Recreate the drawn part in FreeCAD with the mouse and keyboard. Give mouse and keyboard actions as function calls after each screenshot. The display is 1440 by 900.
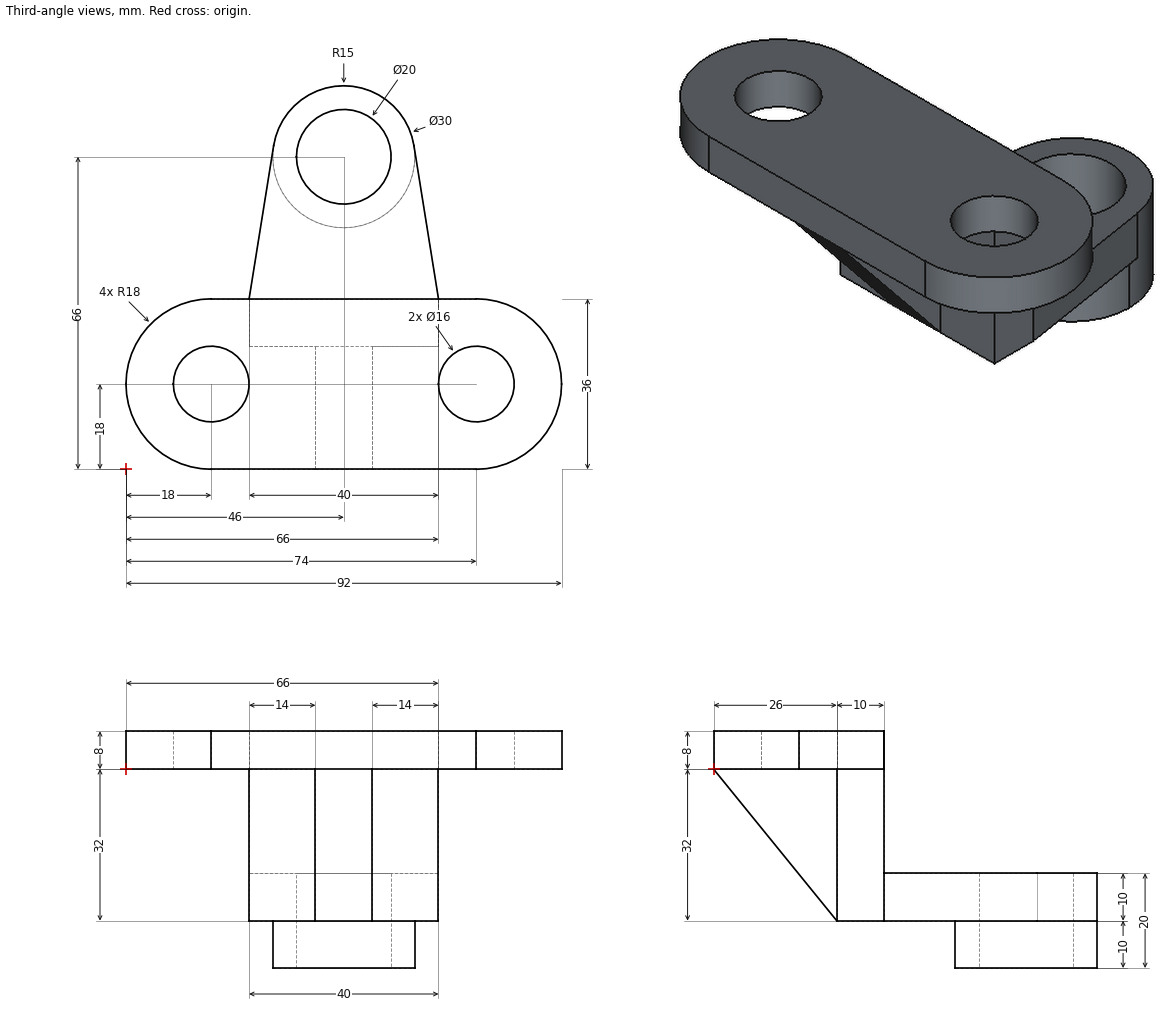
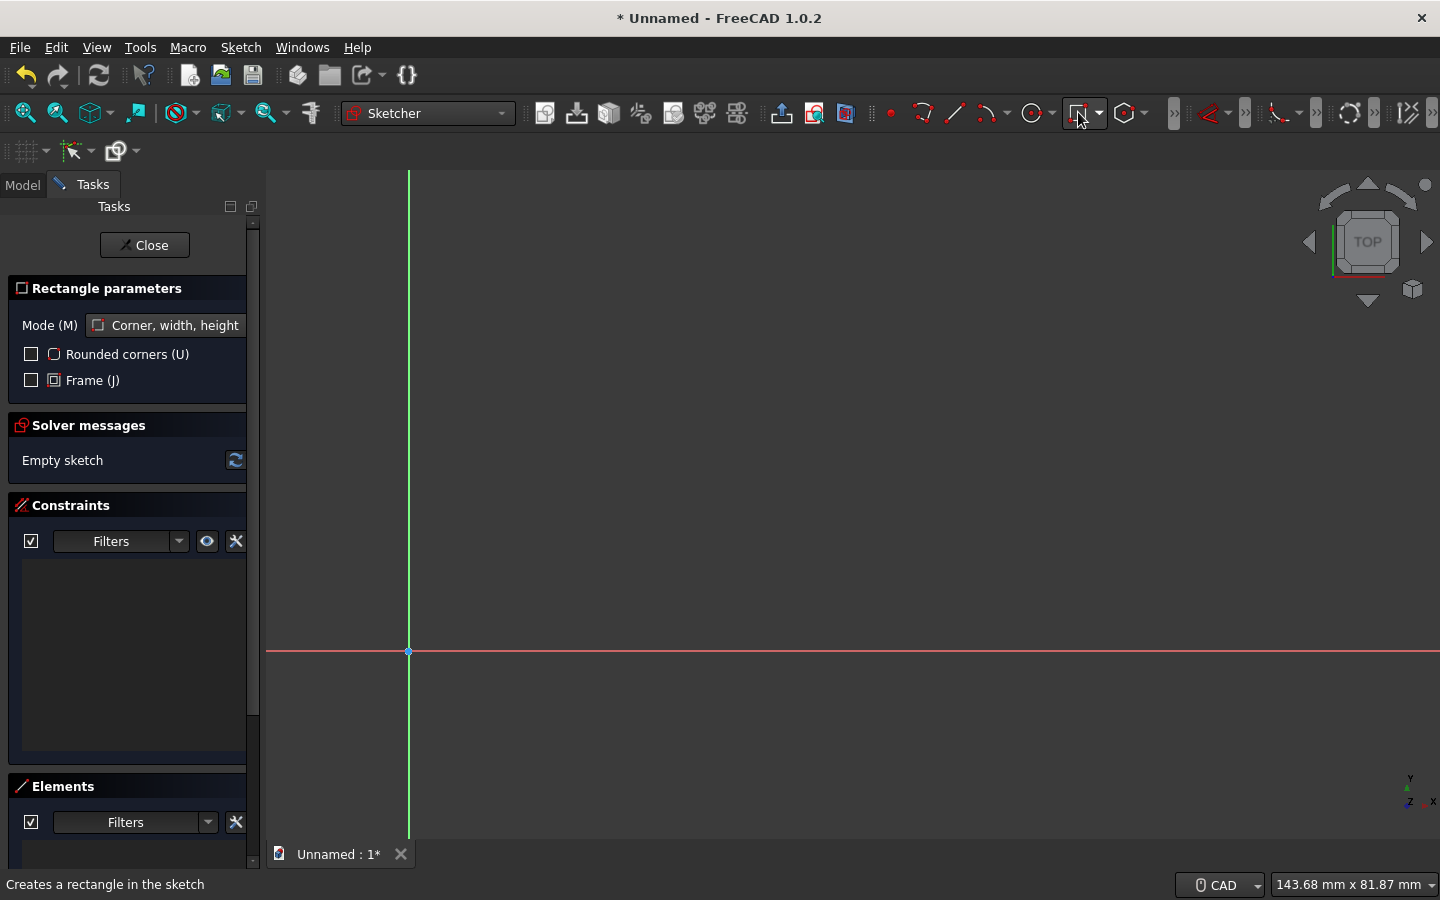
click(409, 651)
move(1160, 357)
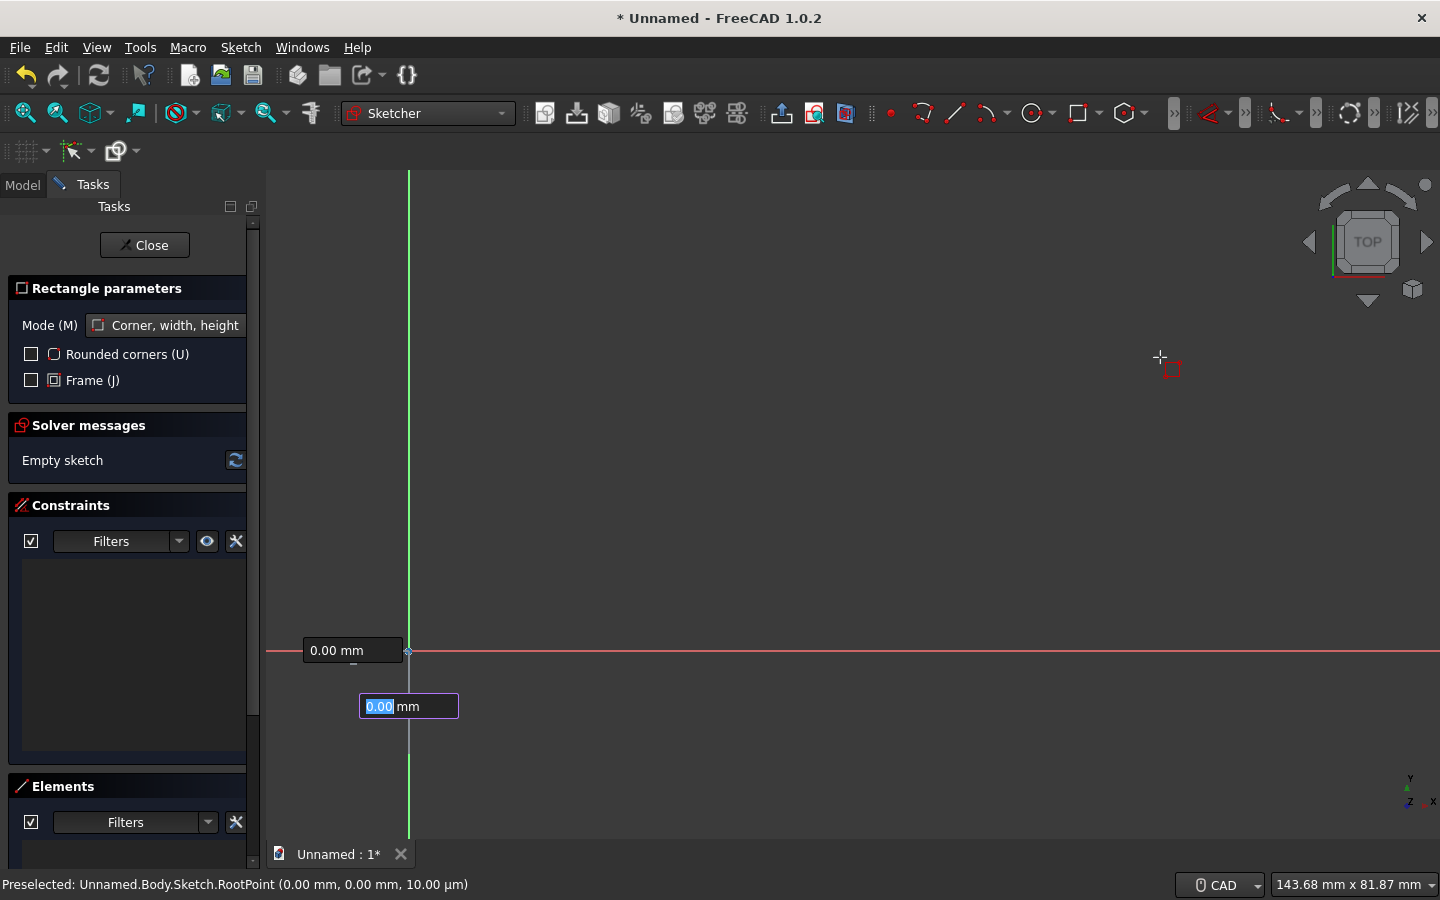
text(92)
key(Tab)
text(36)
key(Return)
key(Escape)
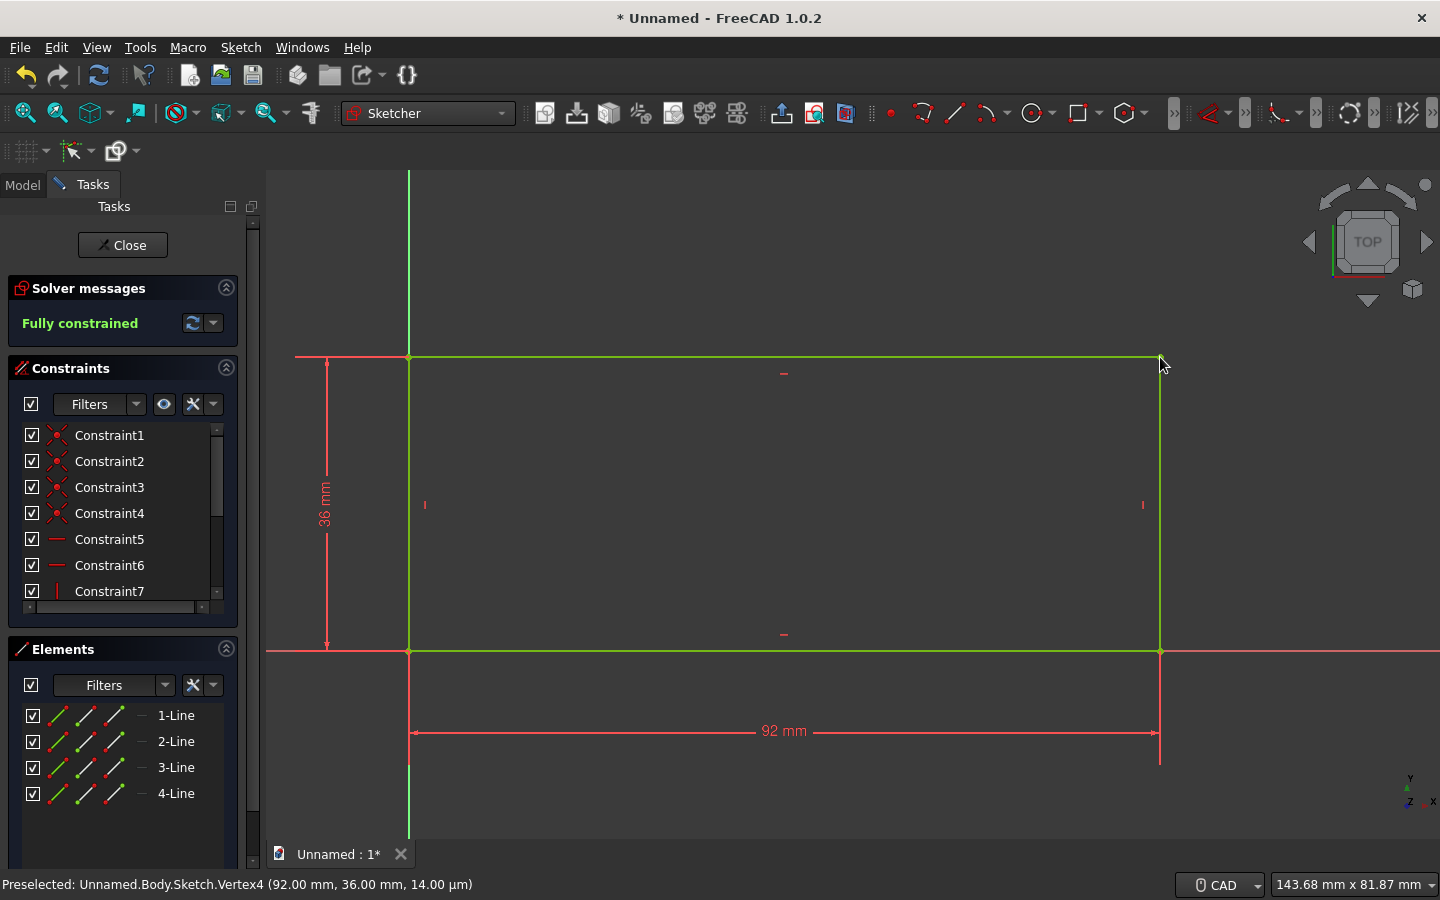
click(123, 245)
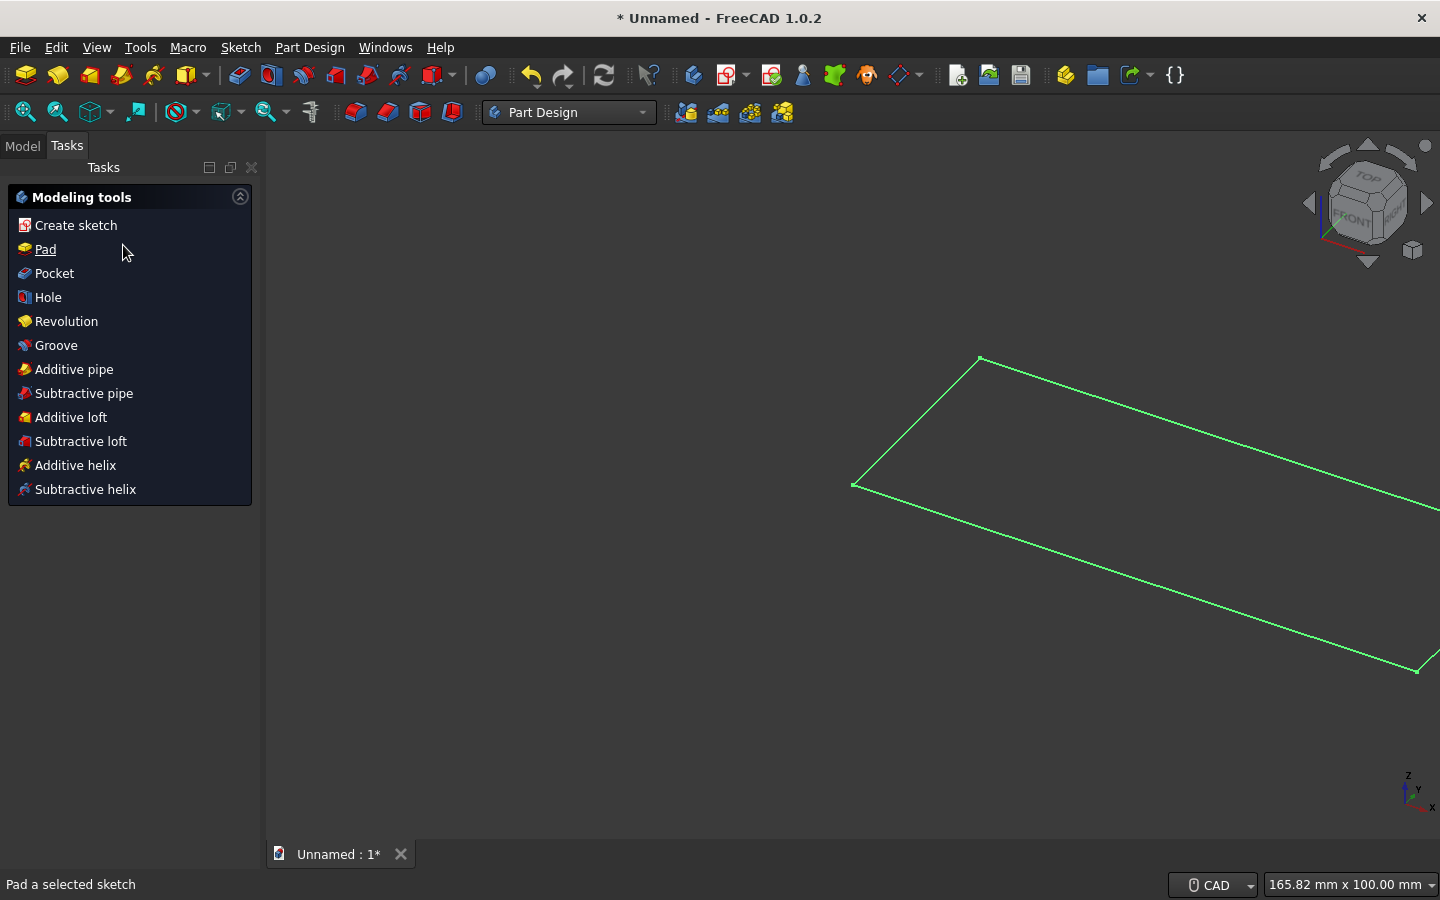
click(26, 76)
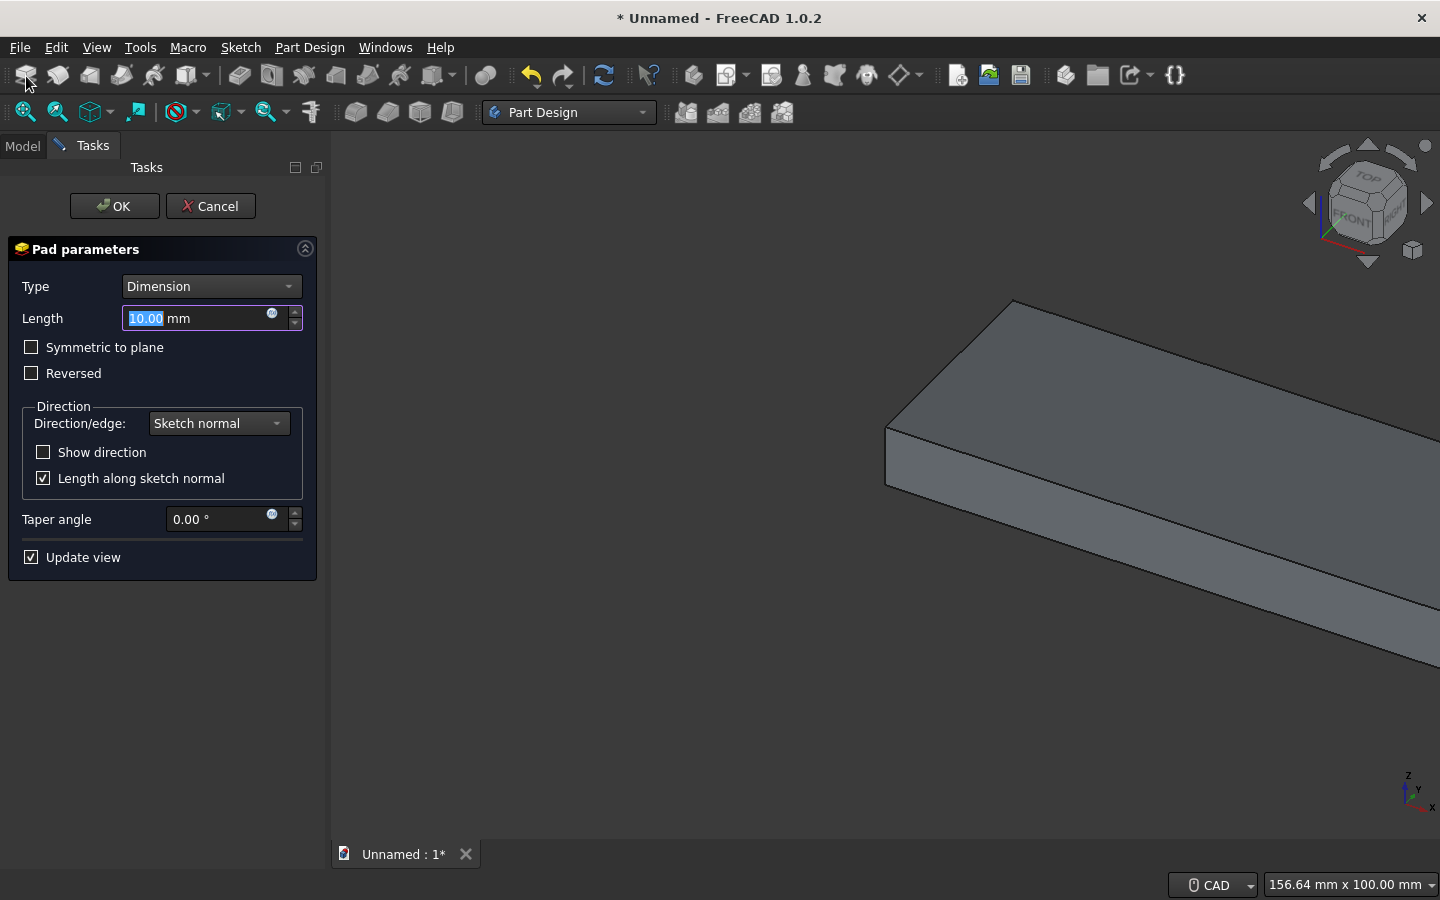
text(8)
key(Tab)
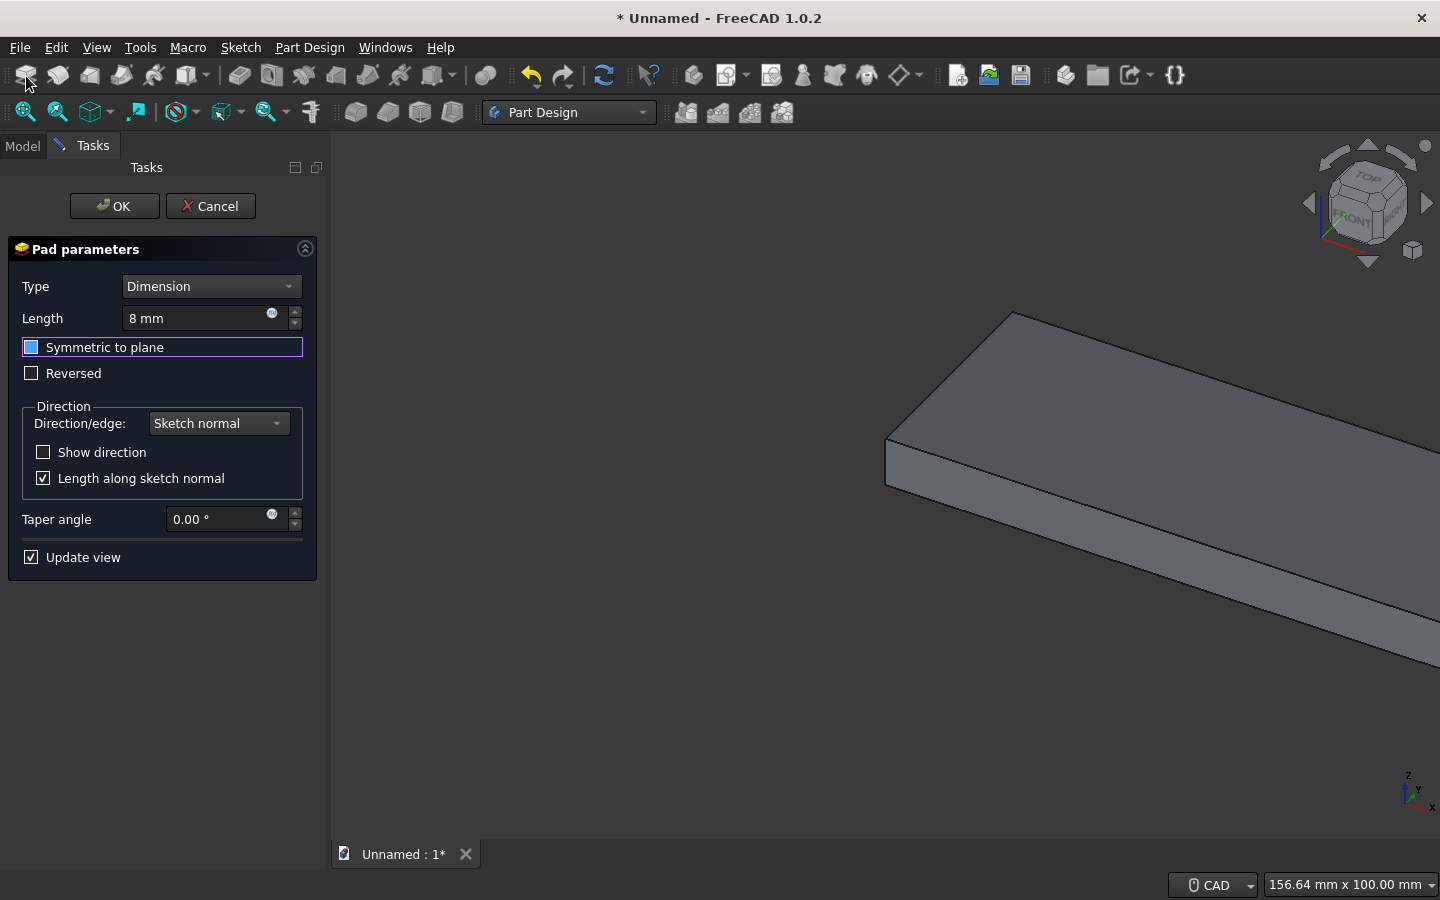
click(115, 206)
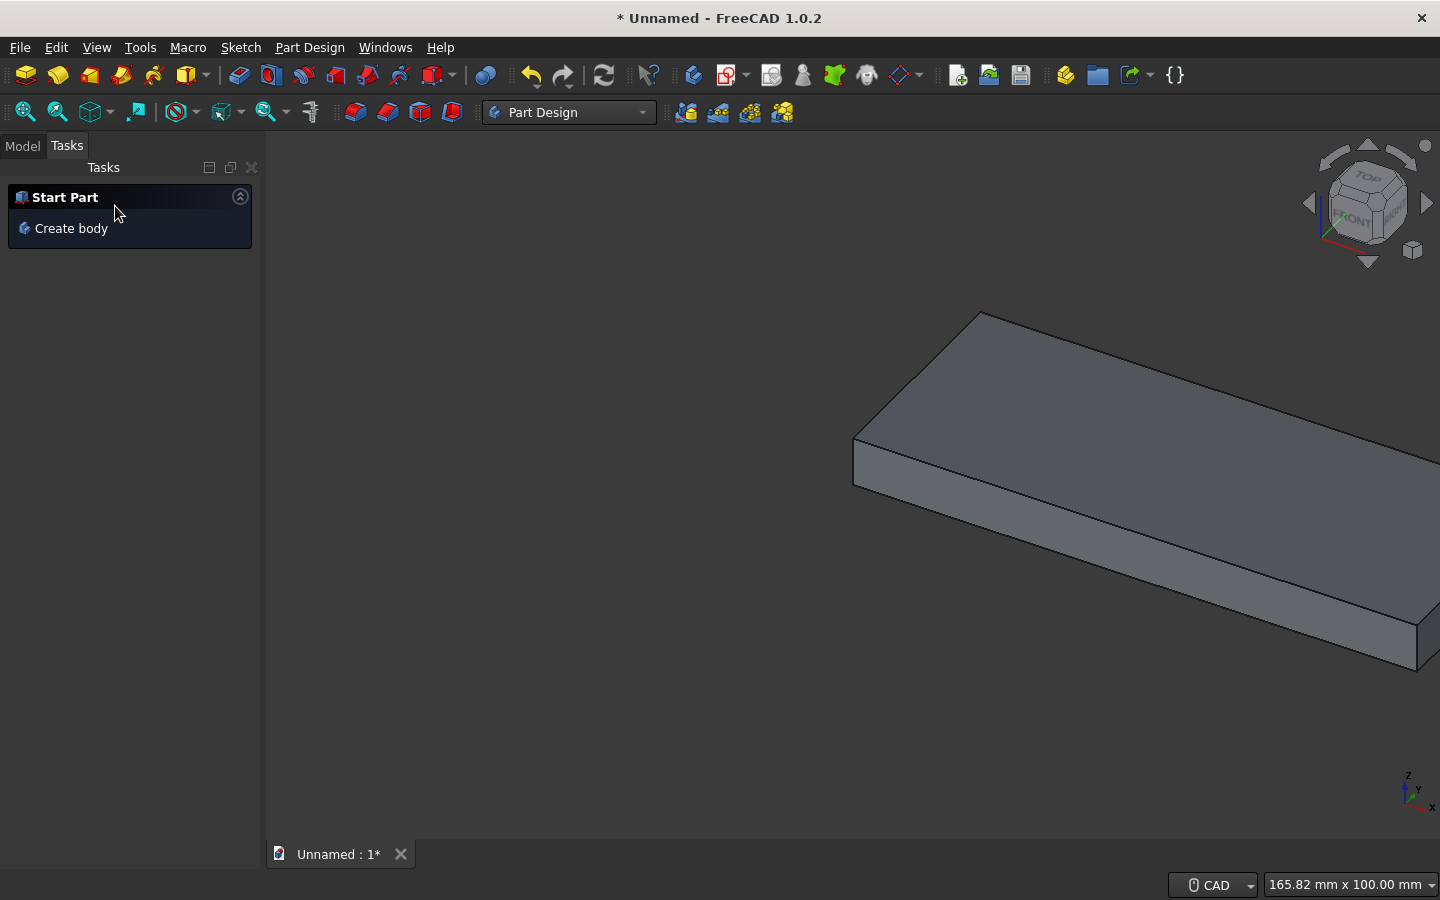
click(26, 112)